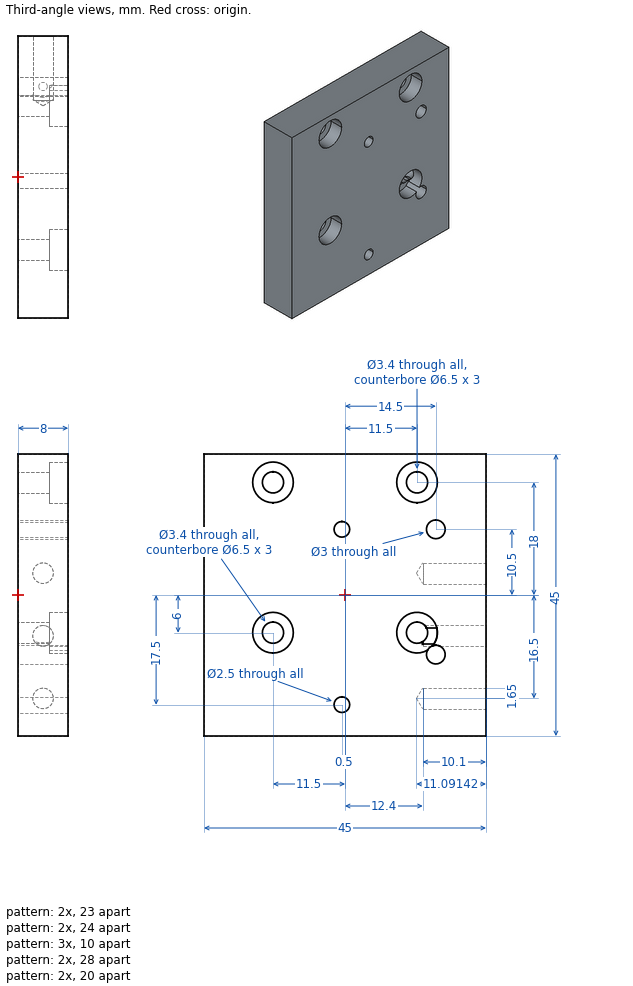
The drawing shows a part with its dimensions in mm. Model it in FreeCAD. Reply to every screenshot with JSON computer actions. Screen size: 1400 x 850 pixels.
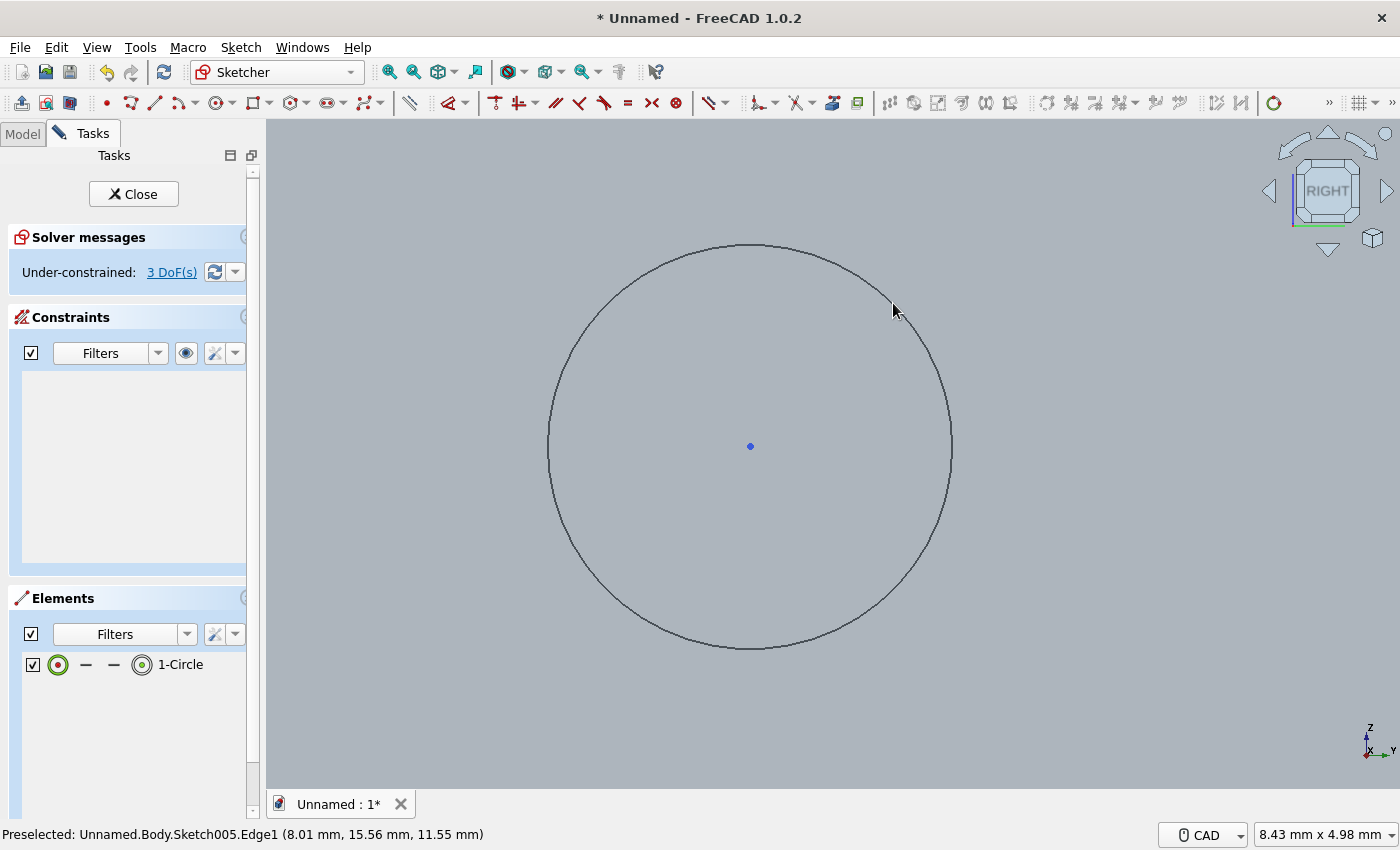
{"action": "key", "text": "d"}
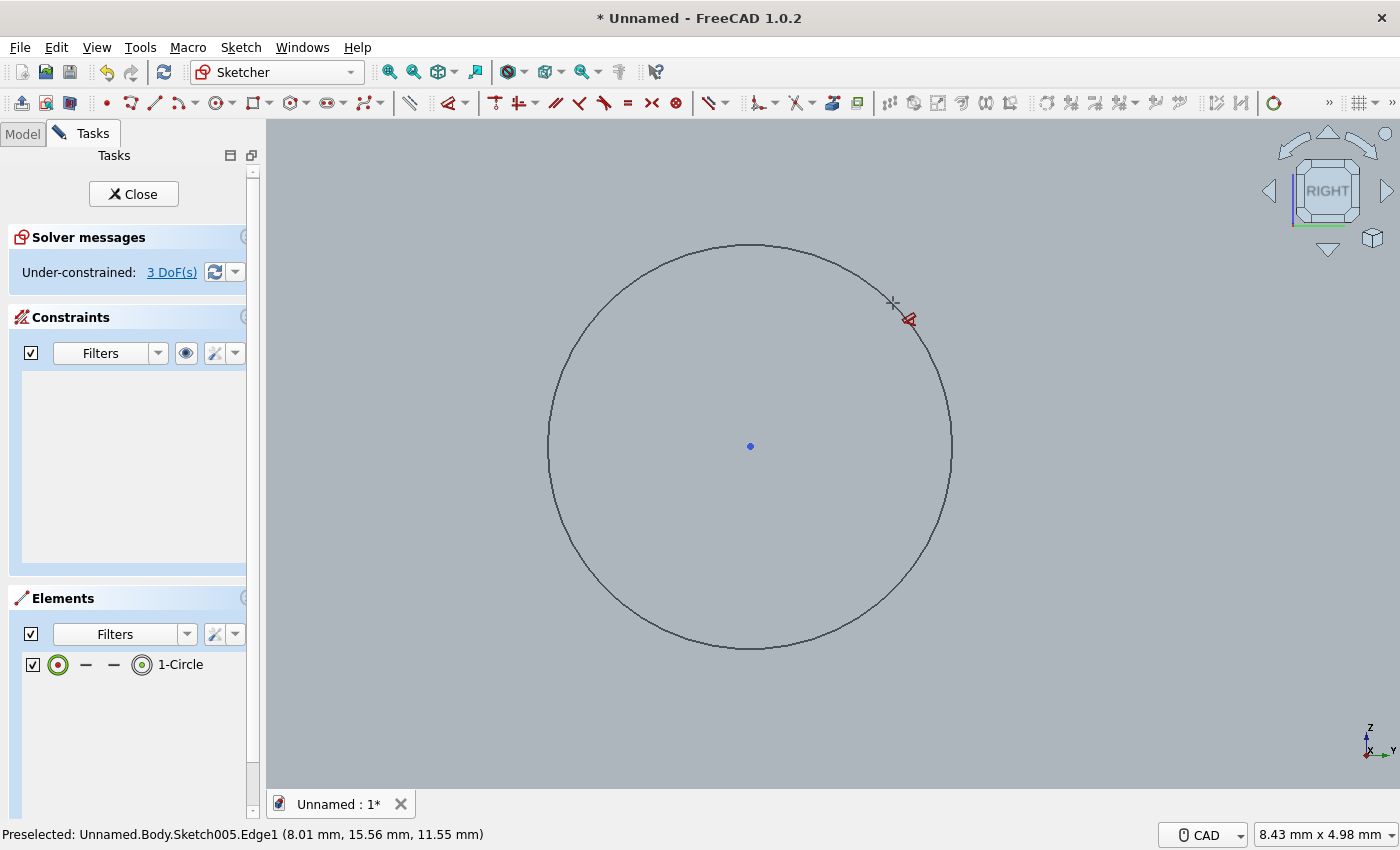
{"action": "left_click", "coordinate": [893, 304]}
{"action": "left_click", "coordinate": [916, 281]}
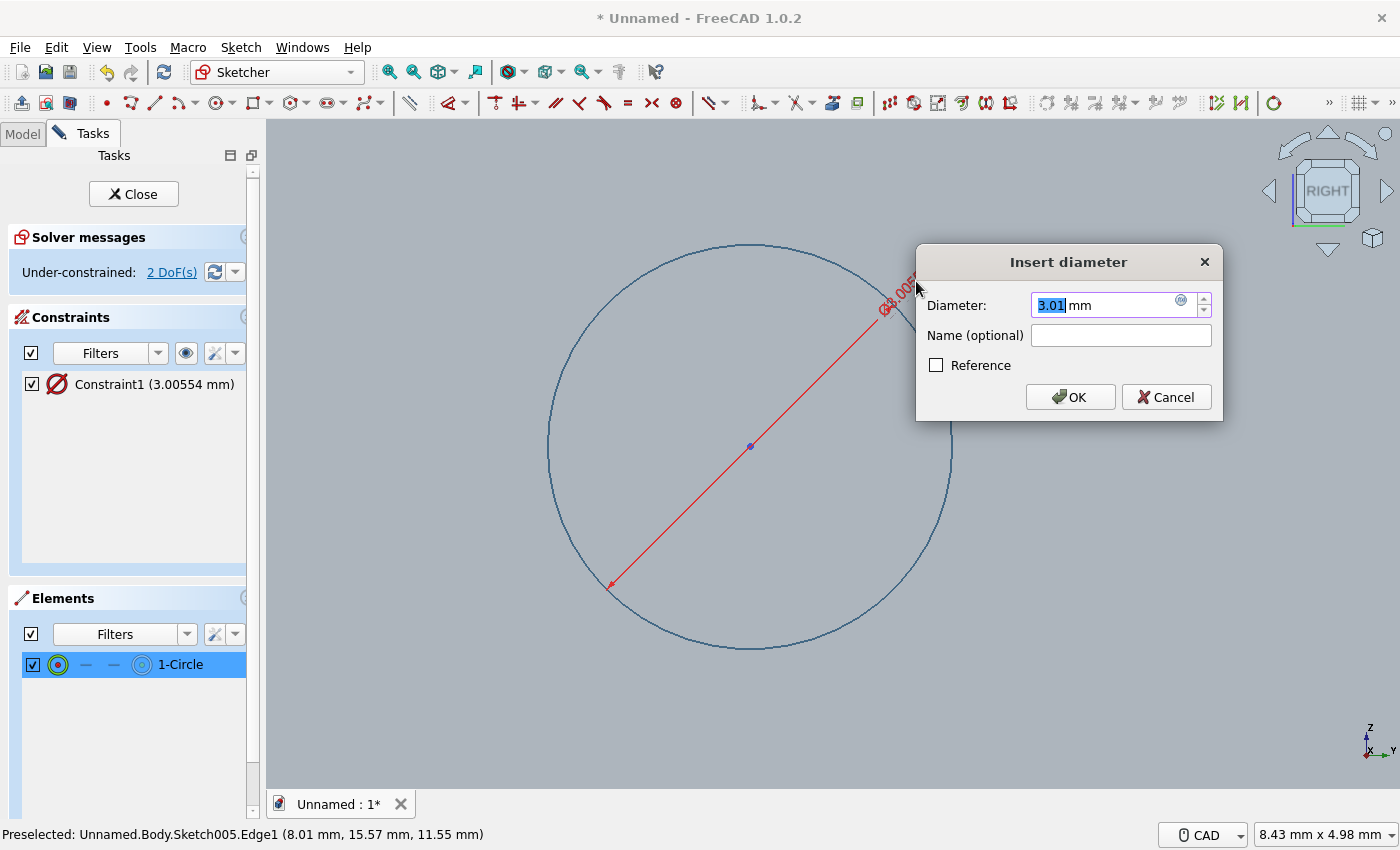
{"action": "type", "text": "3"}
{"action": "key", "text": "Return"}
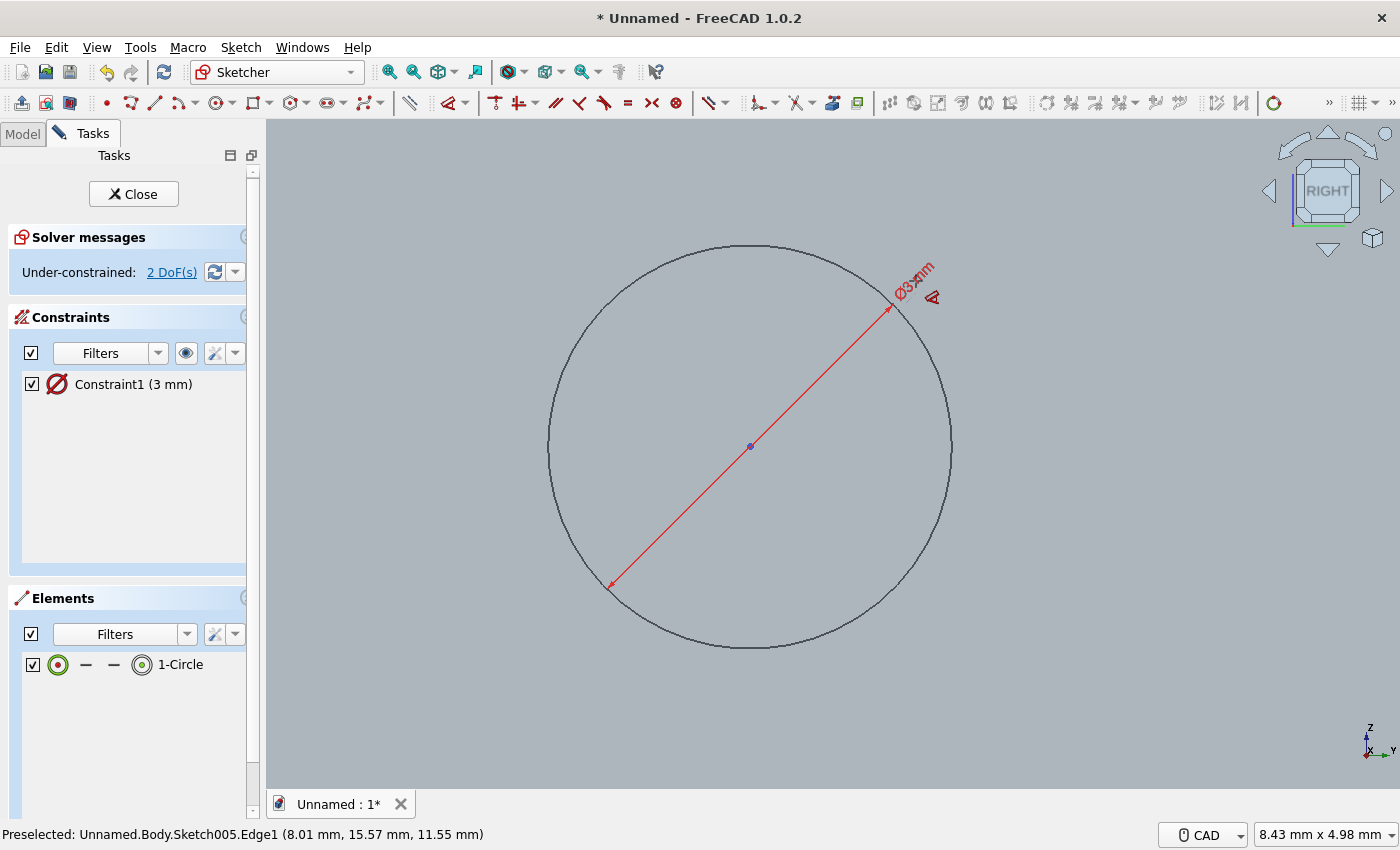
{"action": "left_click", "coordinate": [750, 447]}
{"action": "left_click", "coordinate": [522, 413]}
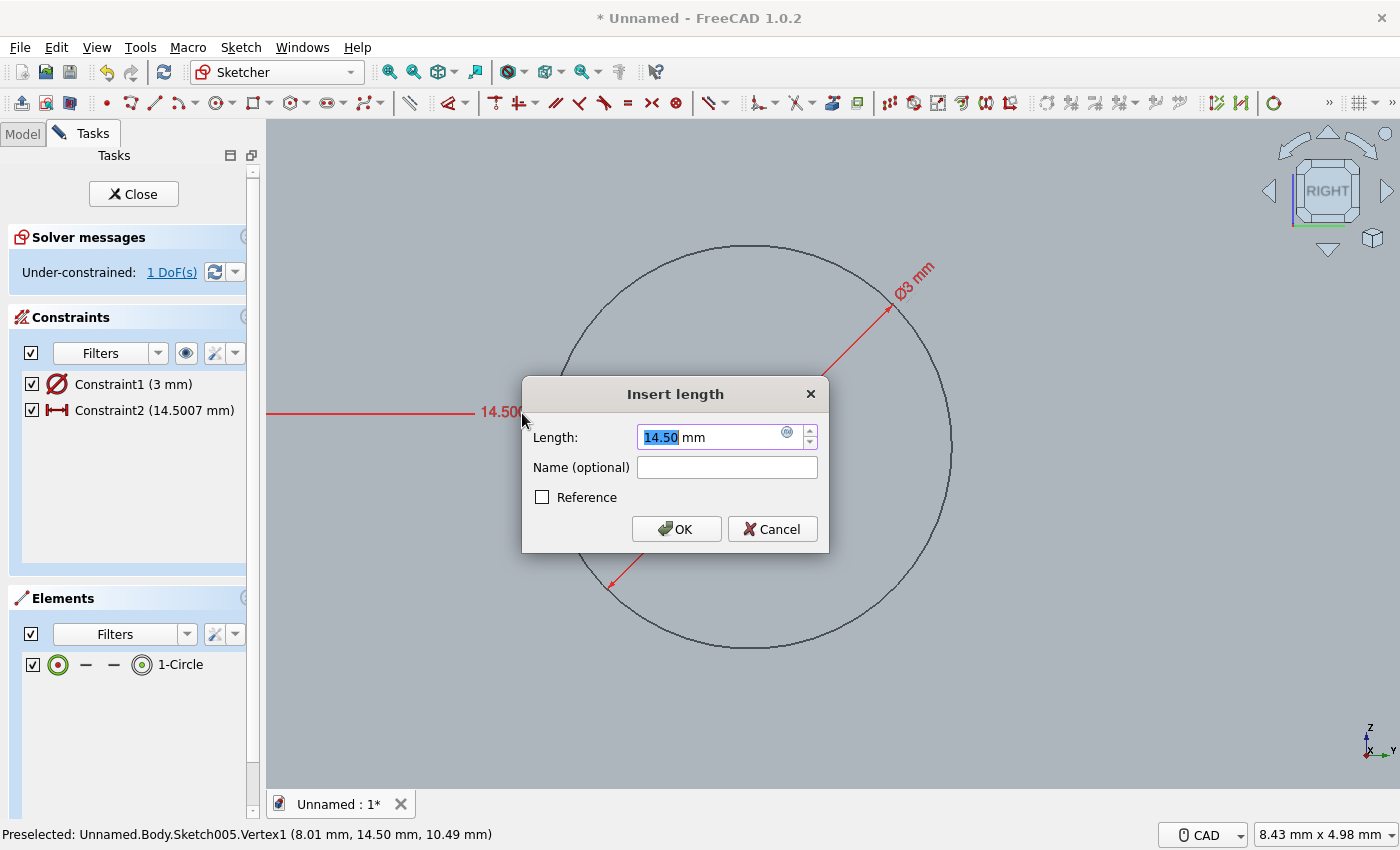
{"action": "type", "text": "14.5"}
{"action": "key", "text": "Return"}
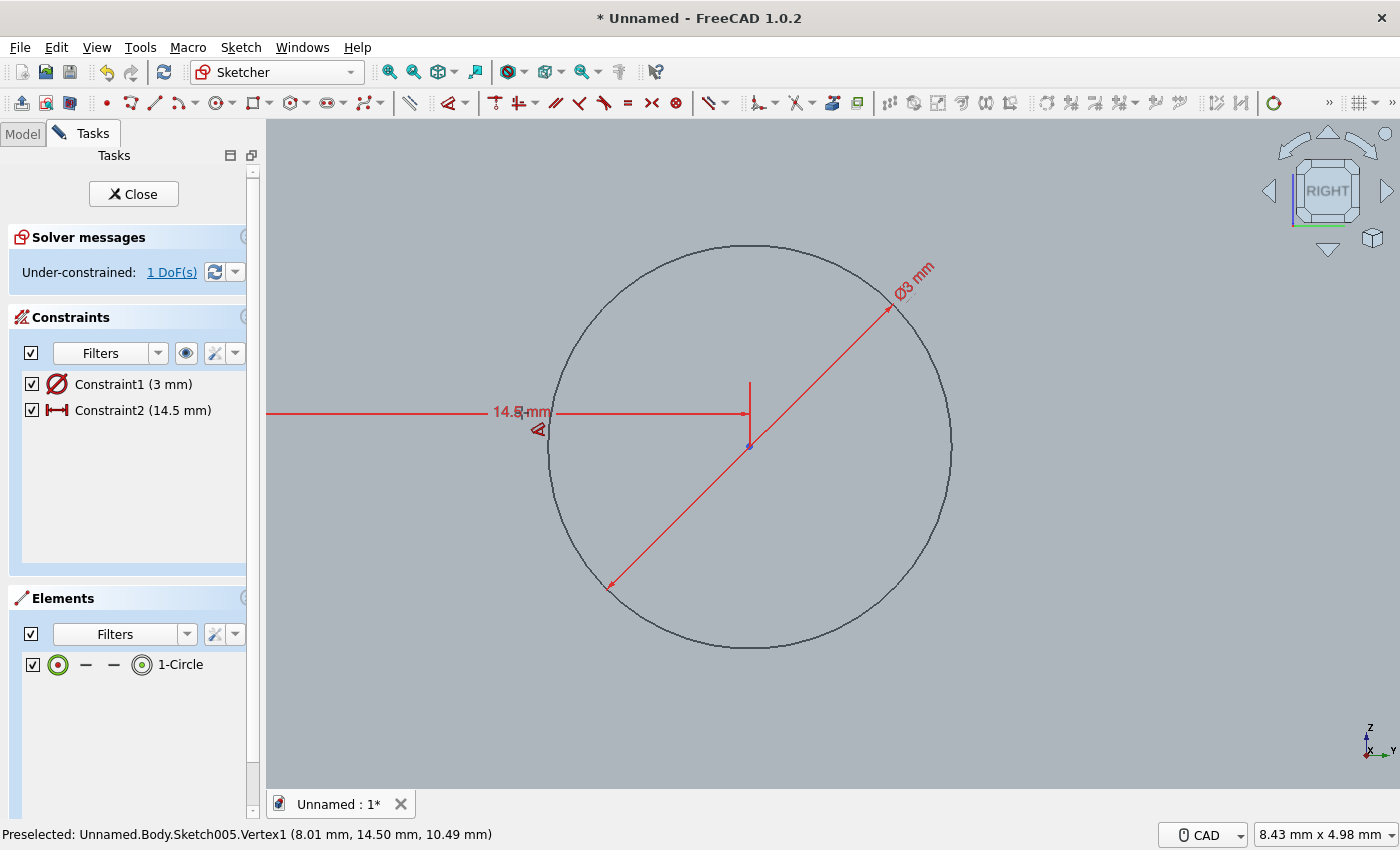
{"action": "left_click", "coordinate": [750, 447]}
{"action": "left_click", "coordinate": [784, 604]}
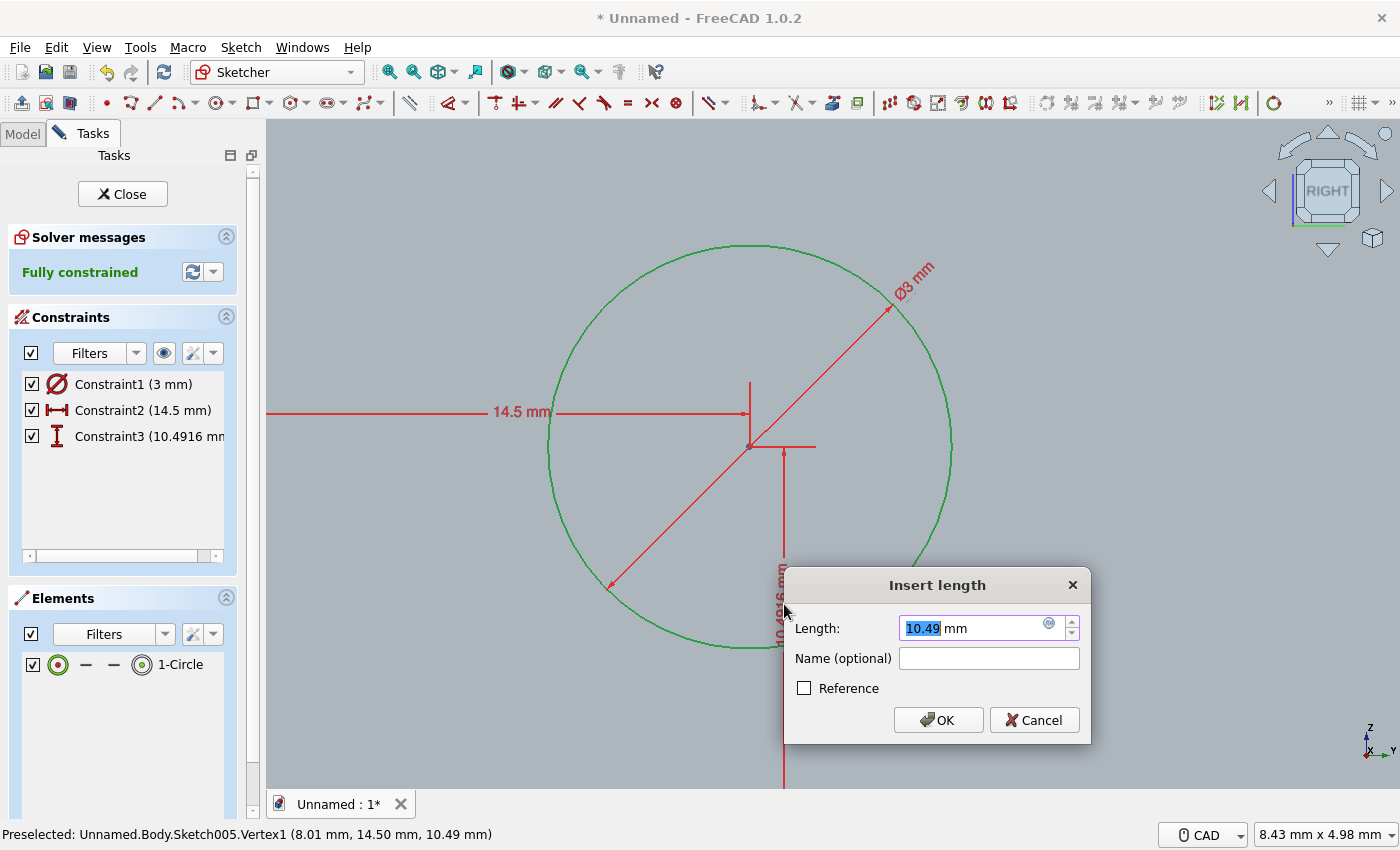
{"action": "type", "text": "10.5"}
{"action": "key", "text": "Return"}
{"action": "key", "text": "Escape"}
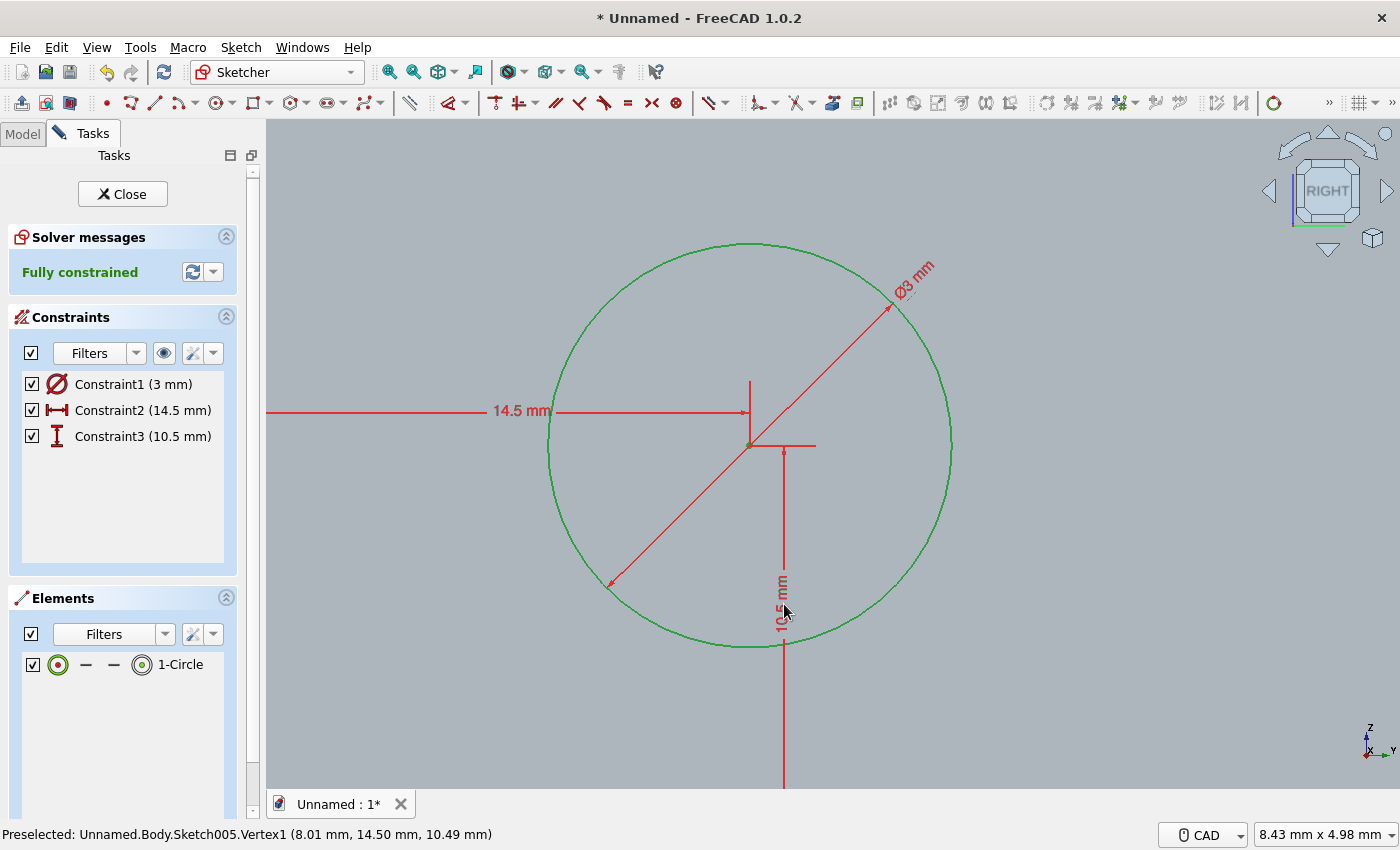
{"action": "left_click", "coordinate": [123, 194]}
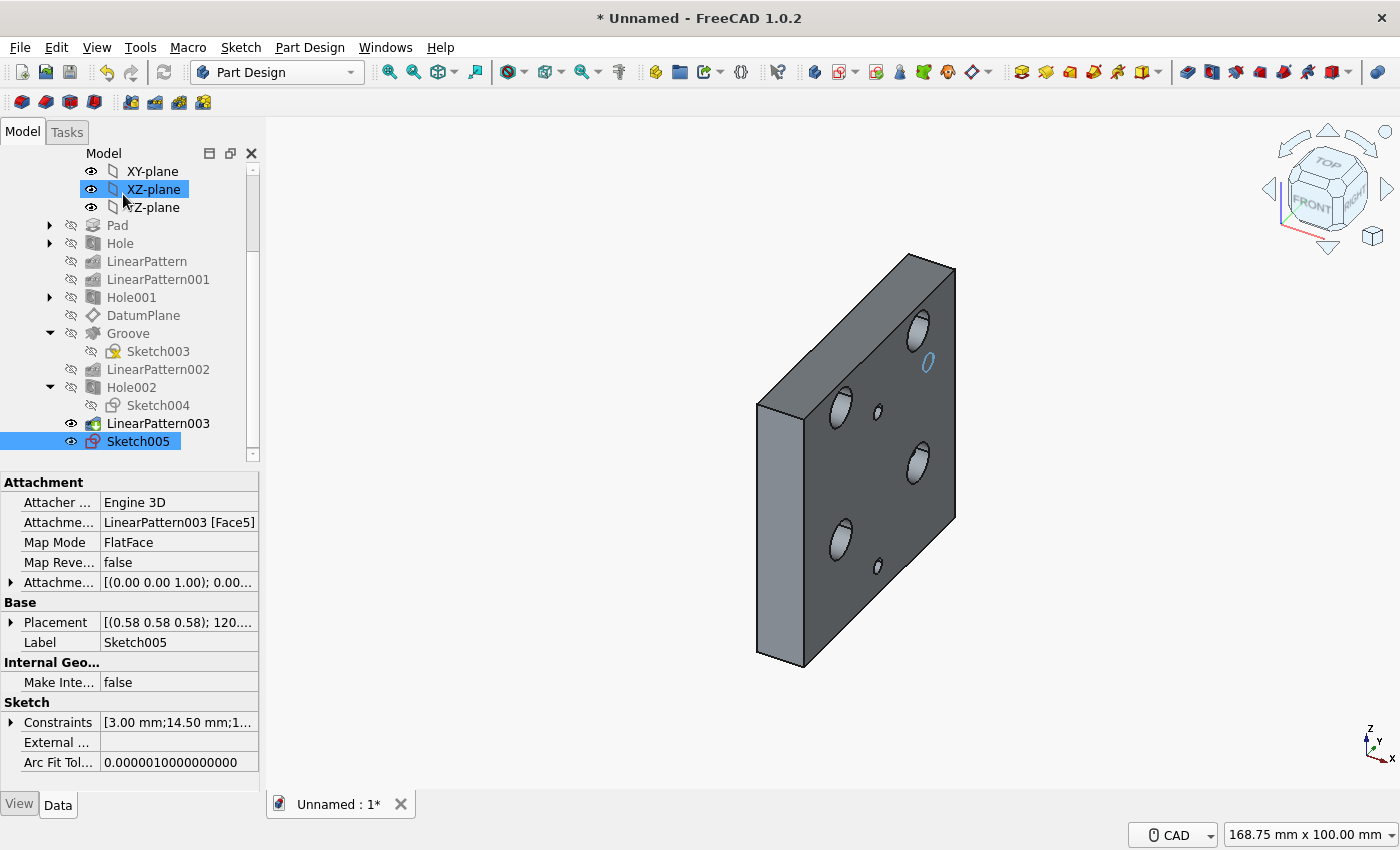
{"action": "left_click", "coordinate": [1212, 72]}